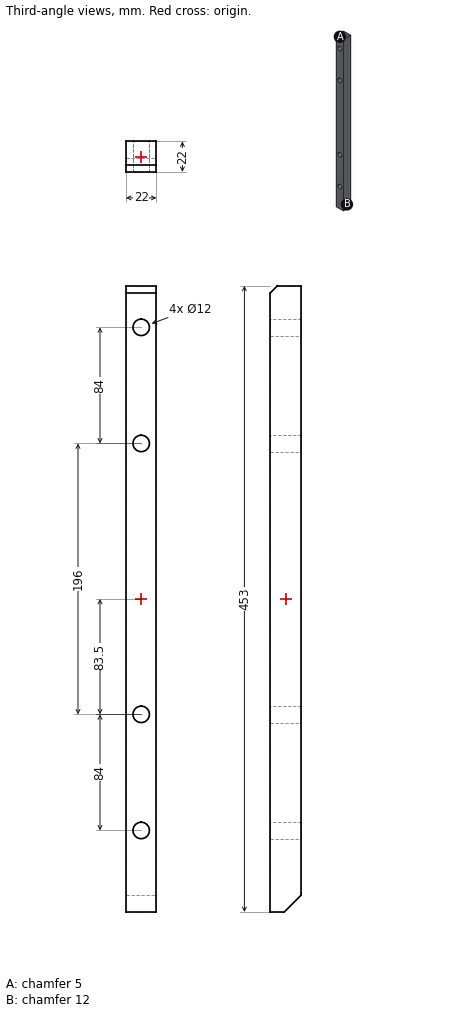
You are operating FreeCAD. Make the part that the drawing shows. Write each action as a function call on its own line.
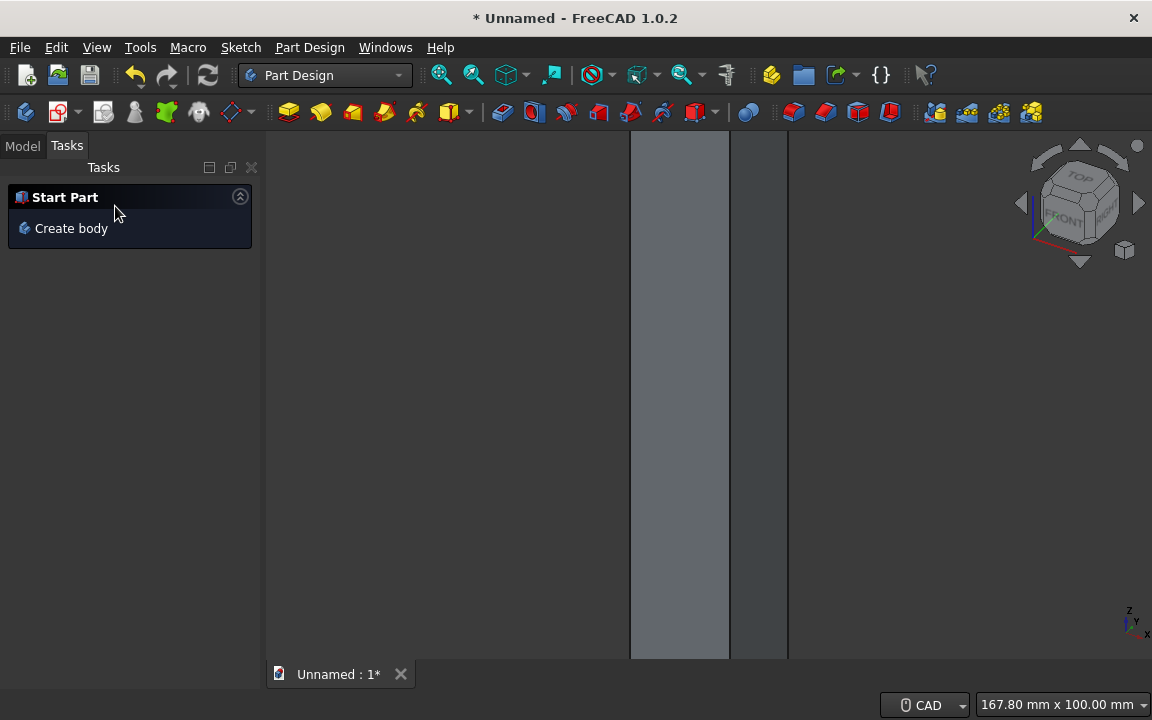
key(v)
key(f)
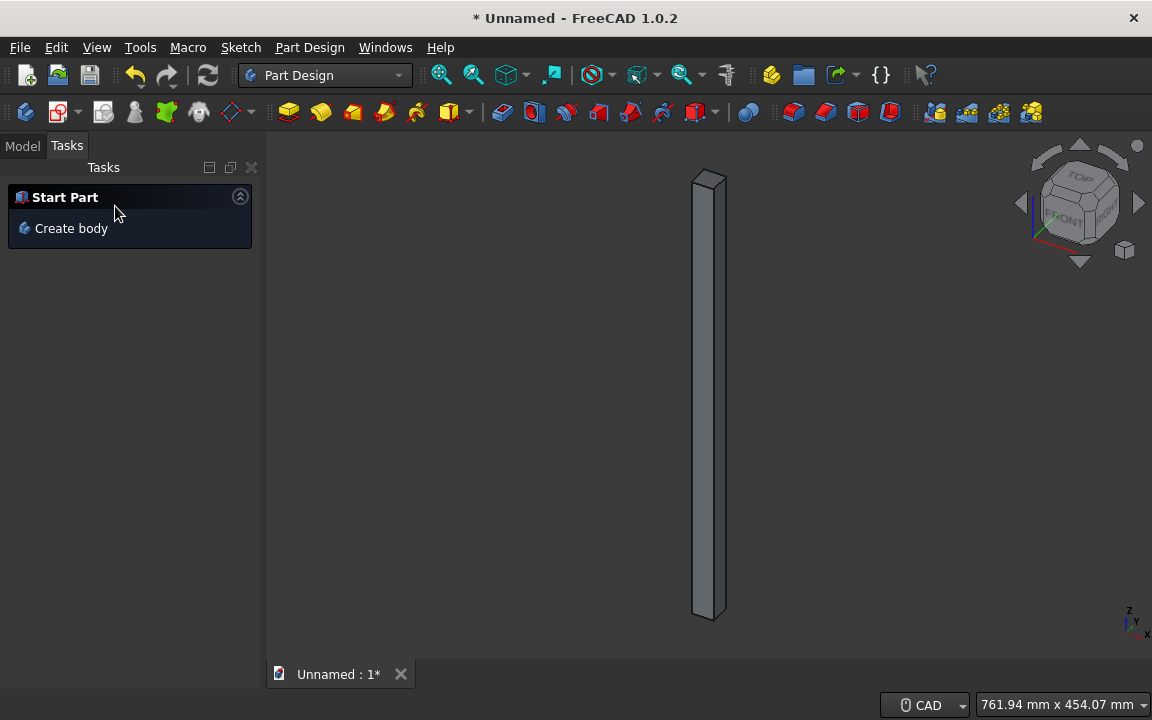
key(4)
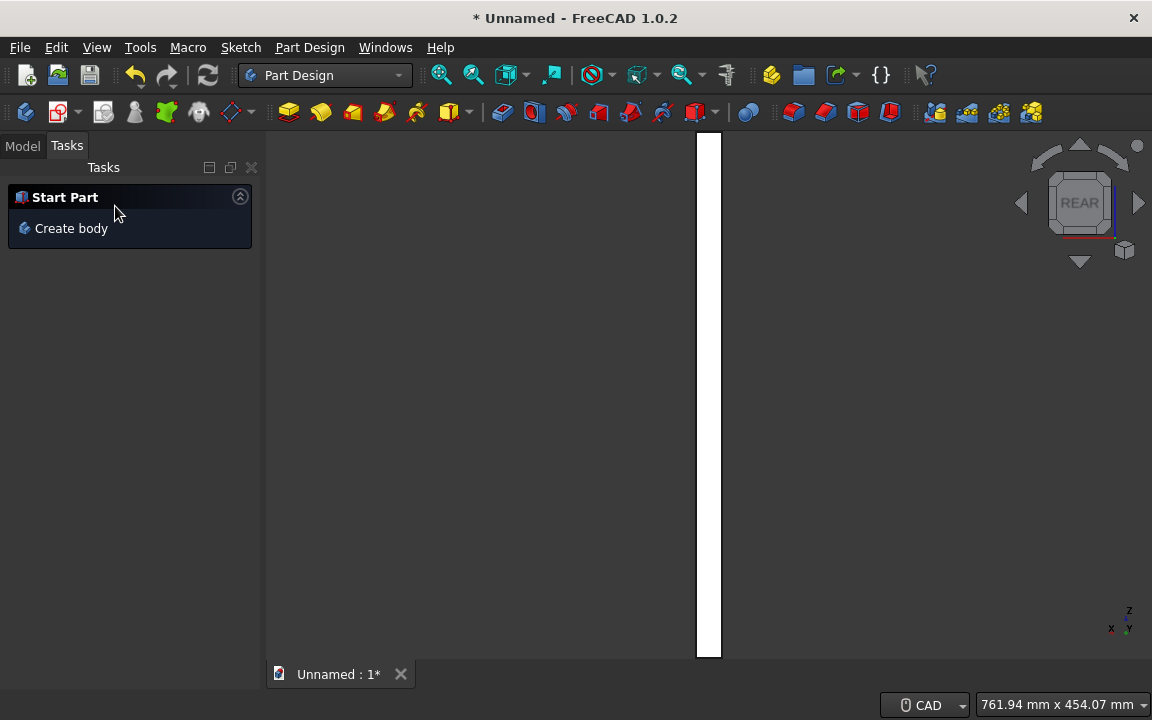
click(709, 168)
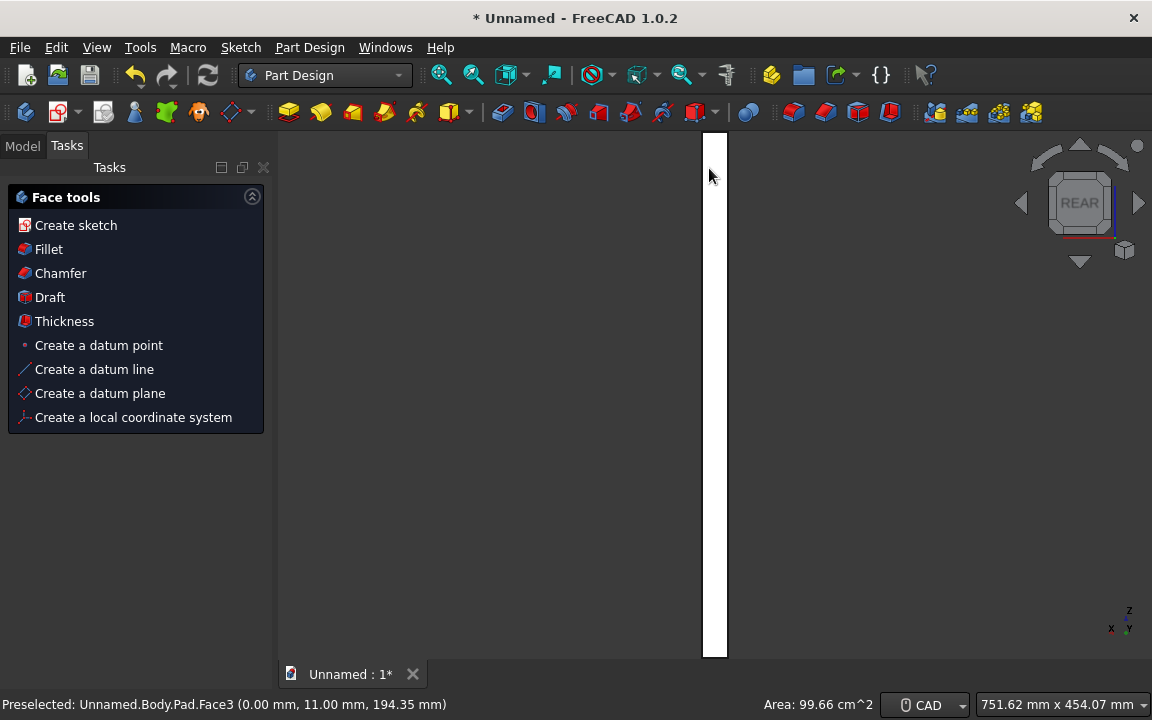
click(58, 112)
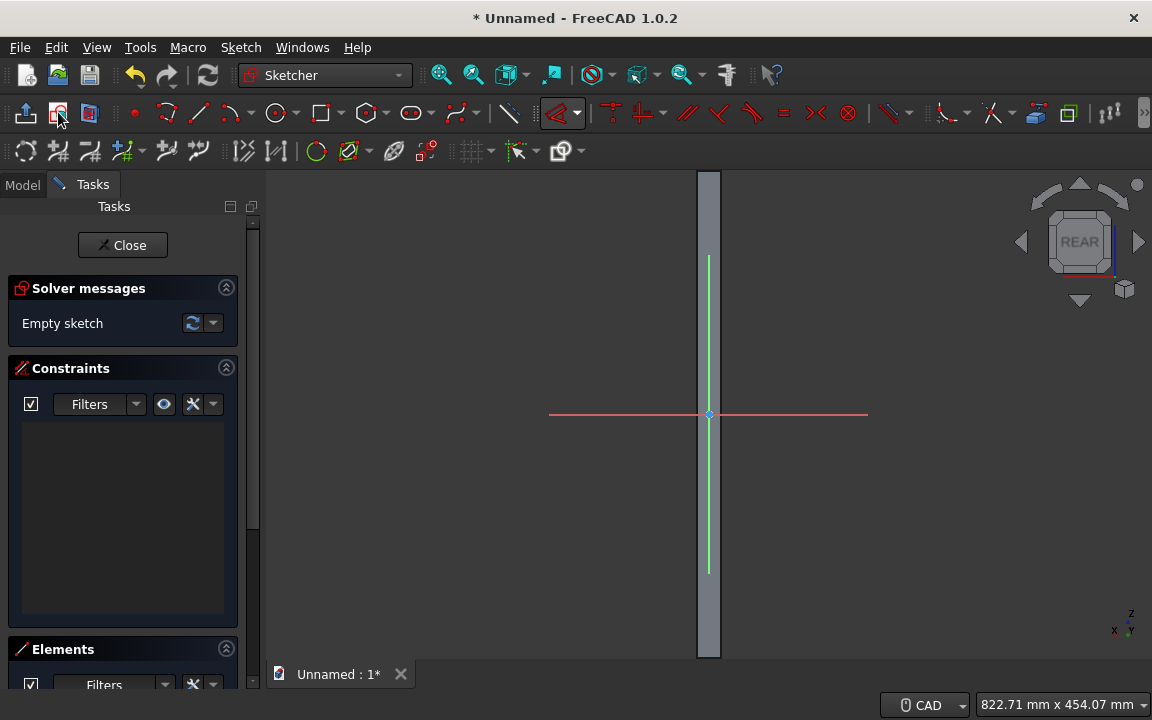
scroll(331, 485, down, 1)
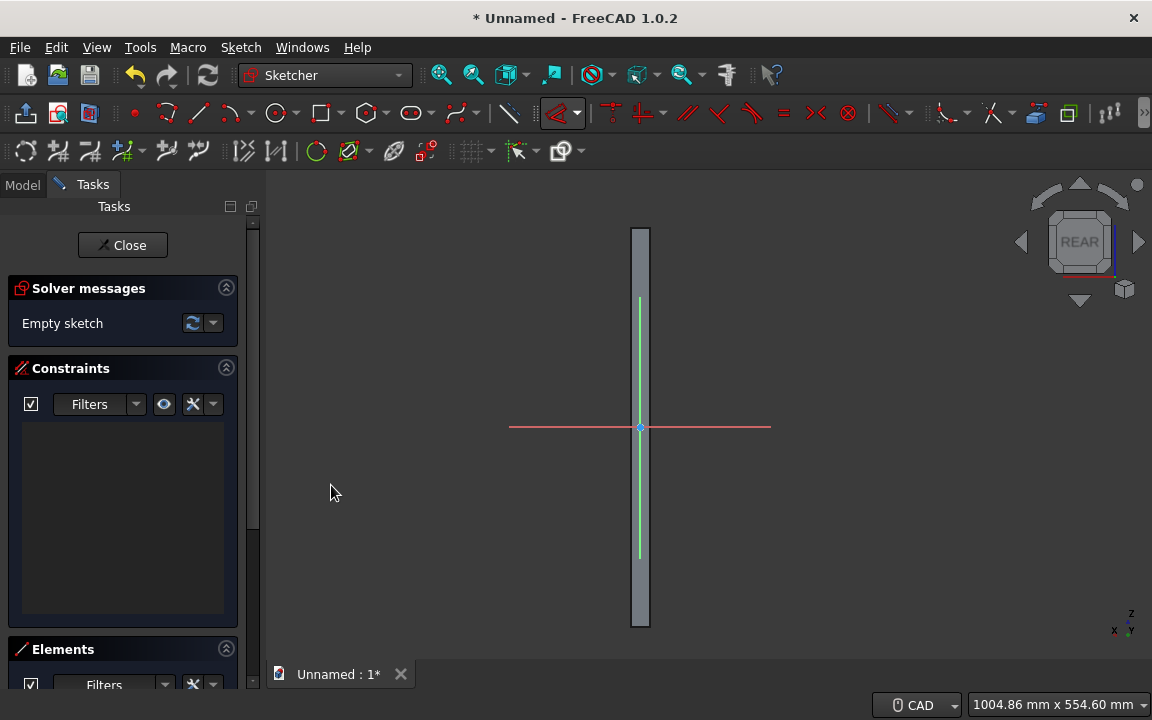
click(276, 114)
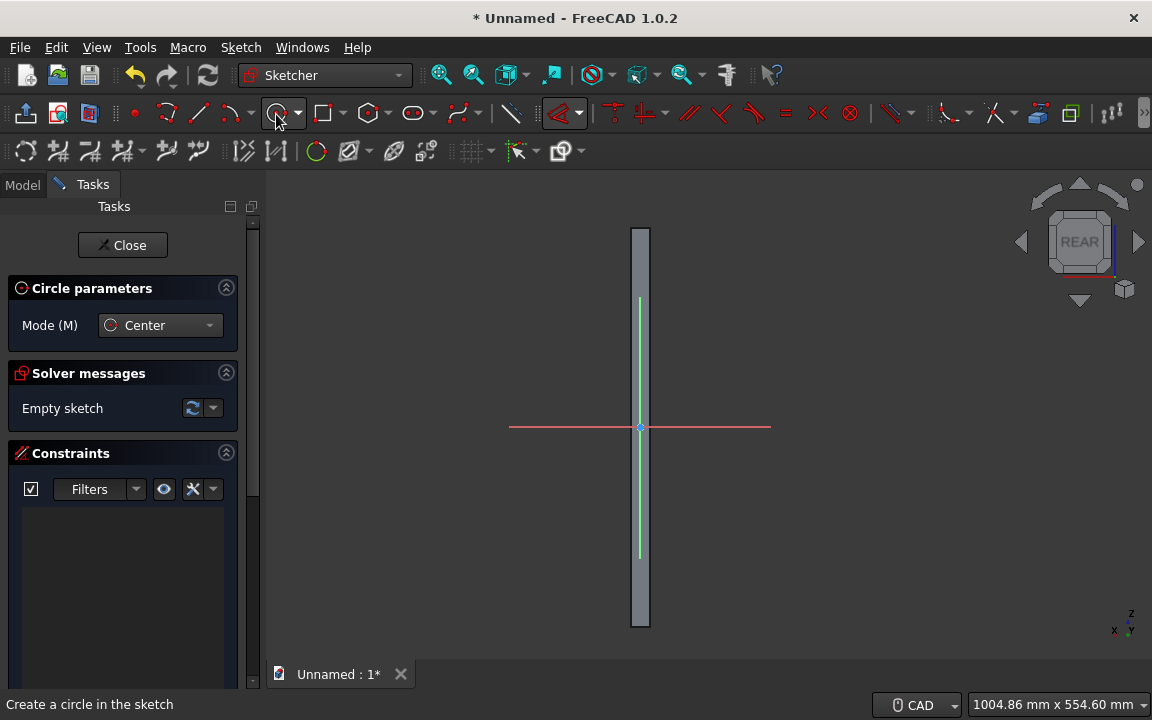
scroll(640, 254, up, 8)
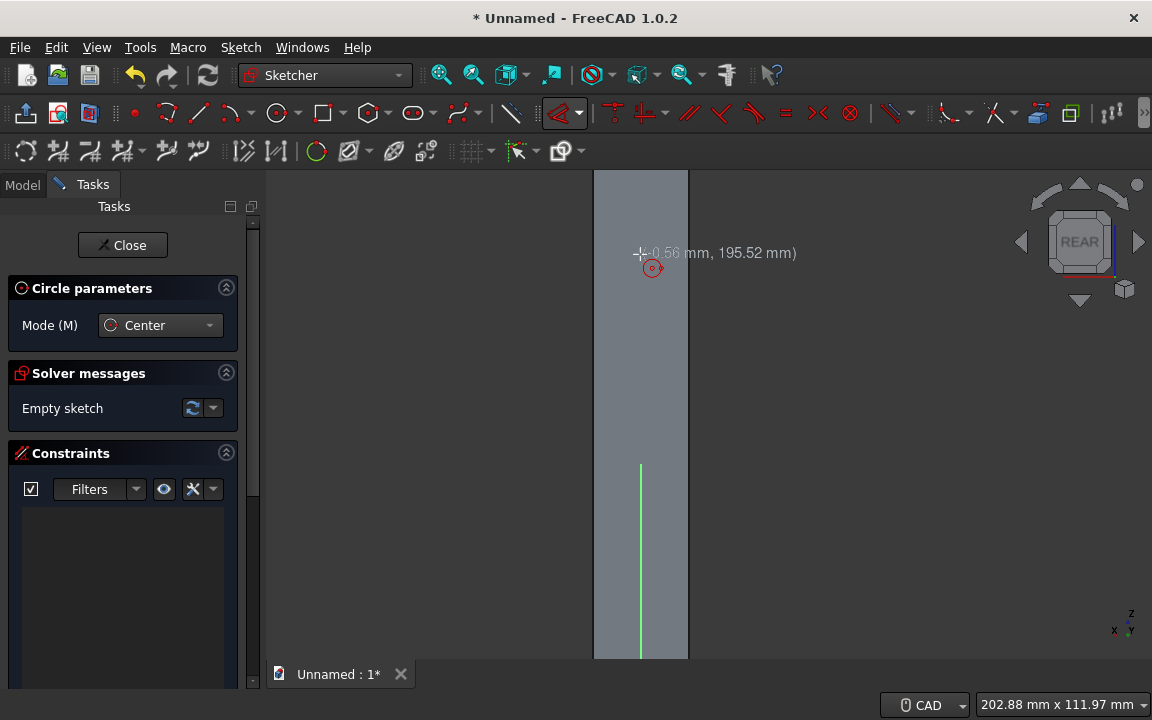
scroll(640, 254, down, 8)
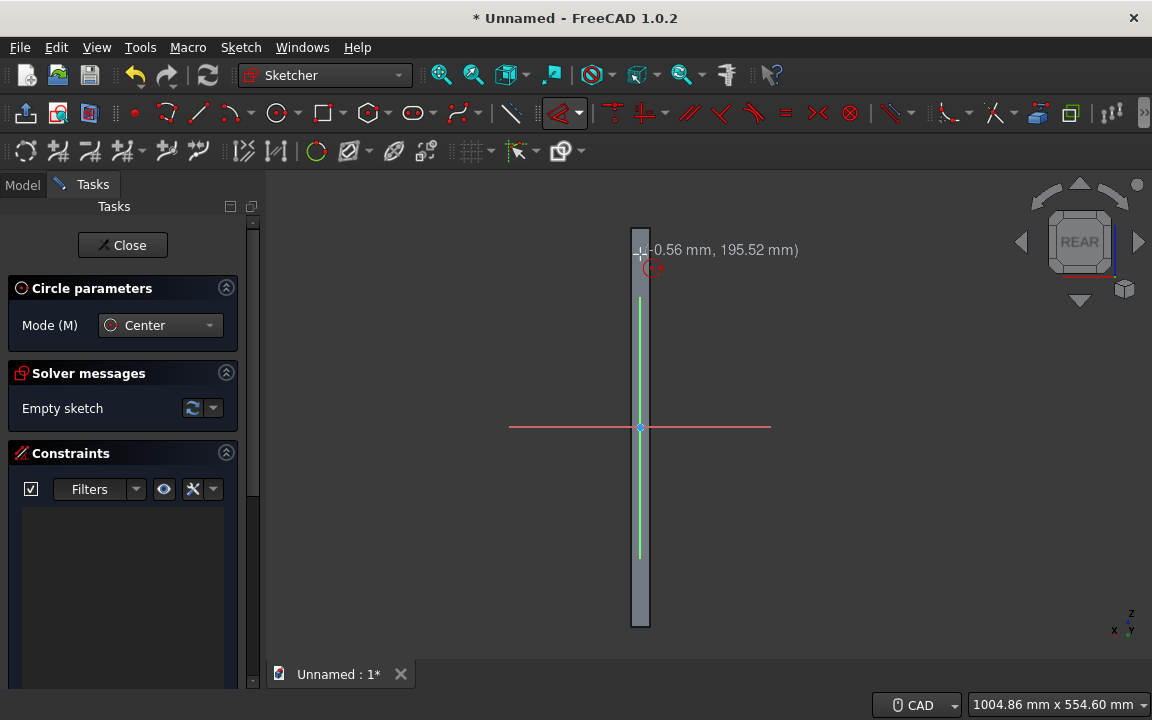
click(640, 254)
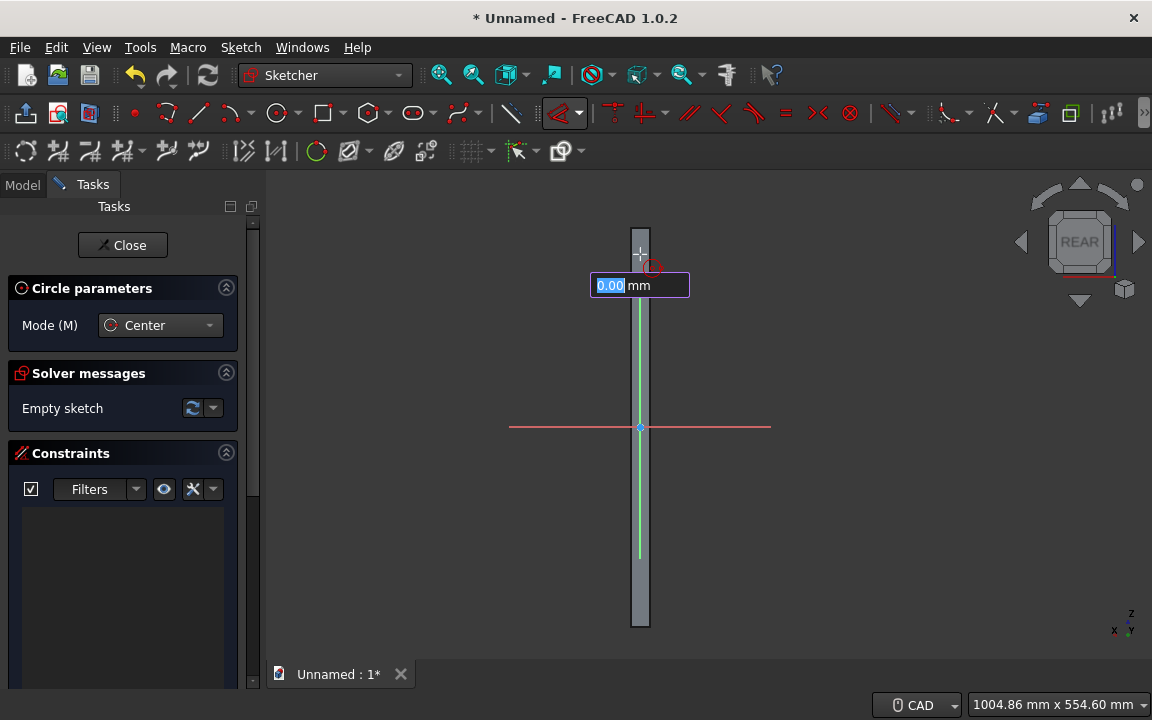
scroll(645, 252, up, 6)
move(646, 253)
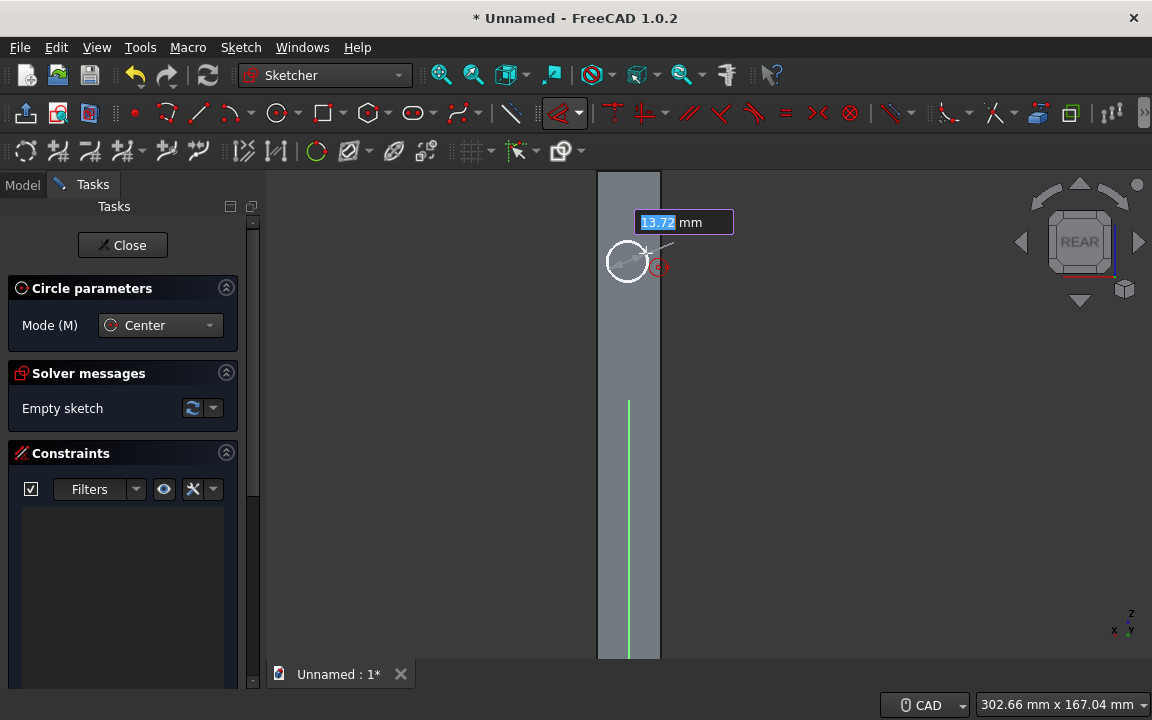
text(12)
key(Return)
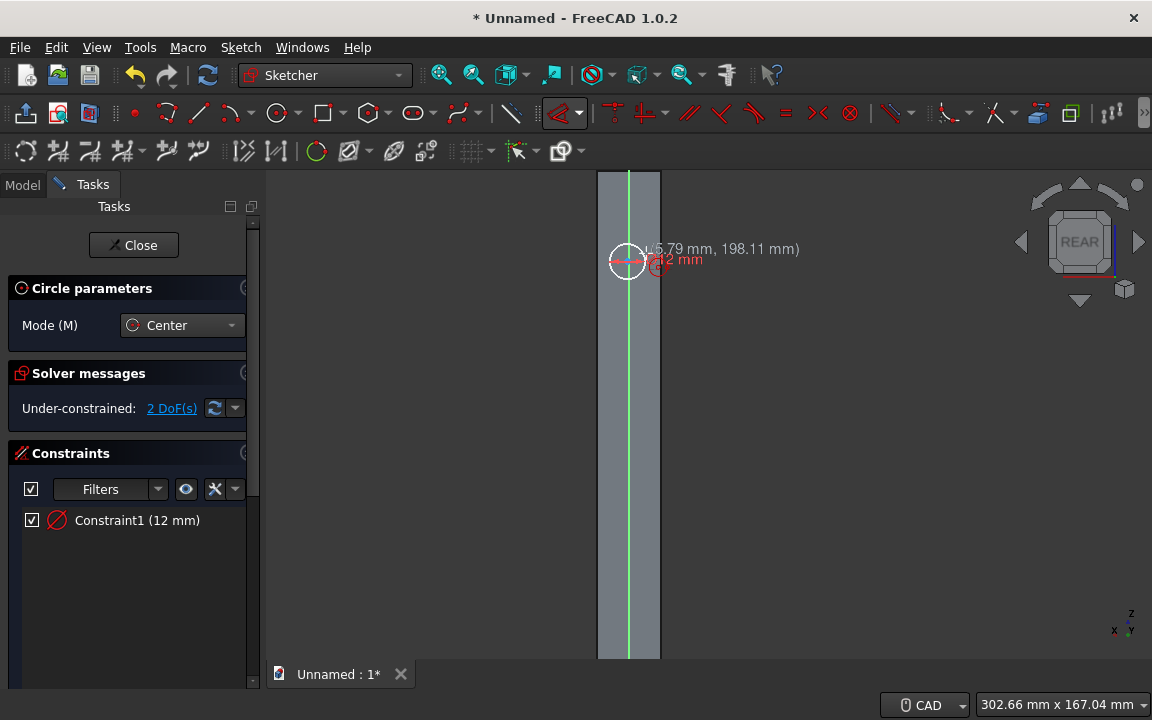
scroll(629, 505, up, 2)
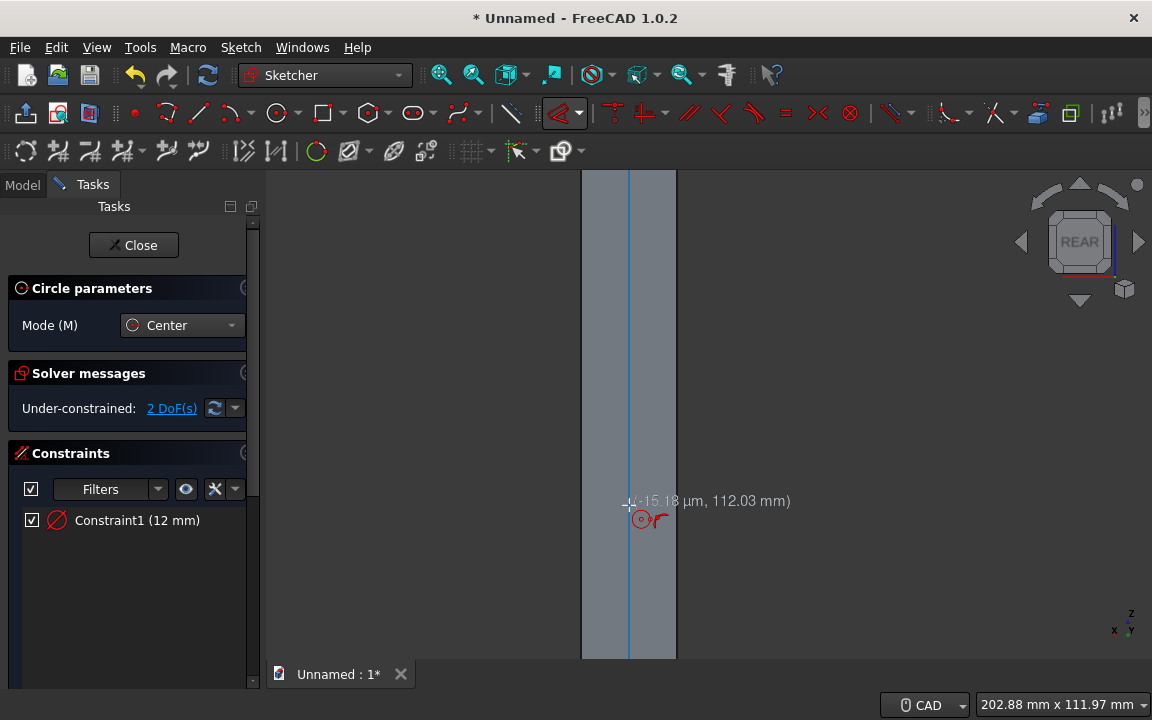
scroll(643, 284, down, 8)